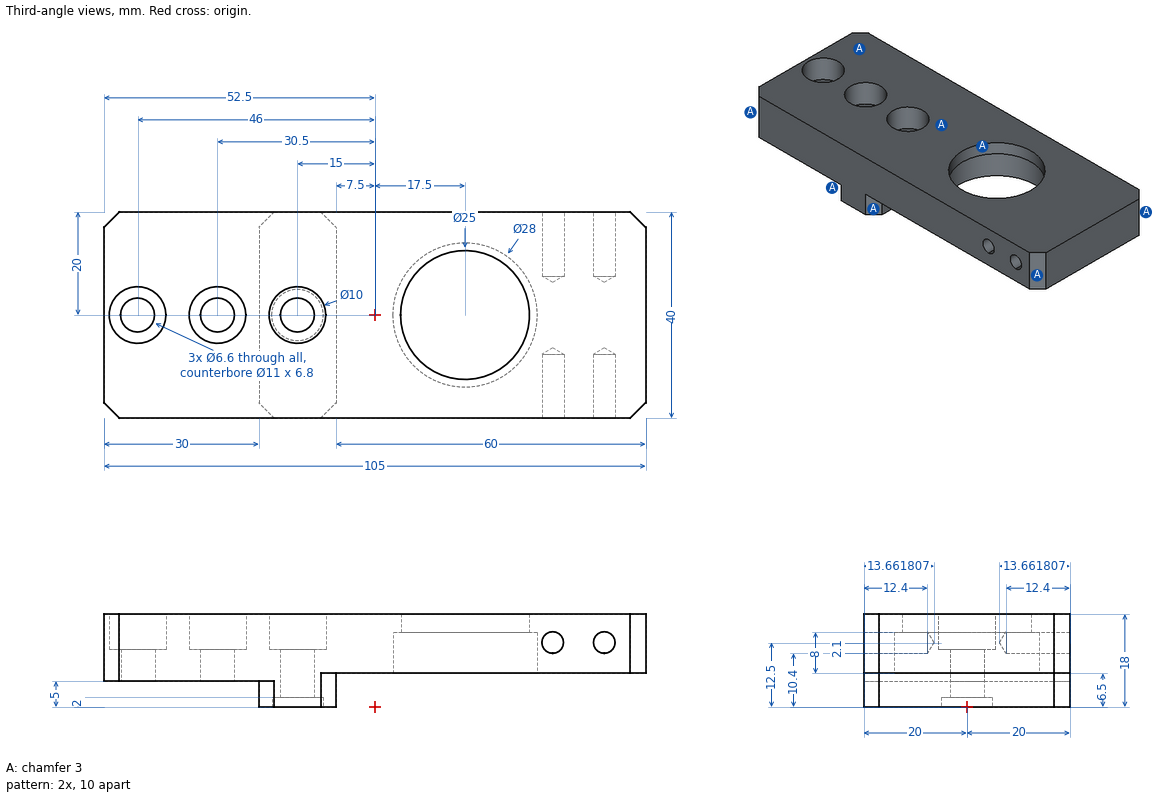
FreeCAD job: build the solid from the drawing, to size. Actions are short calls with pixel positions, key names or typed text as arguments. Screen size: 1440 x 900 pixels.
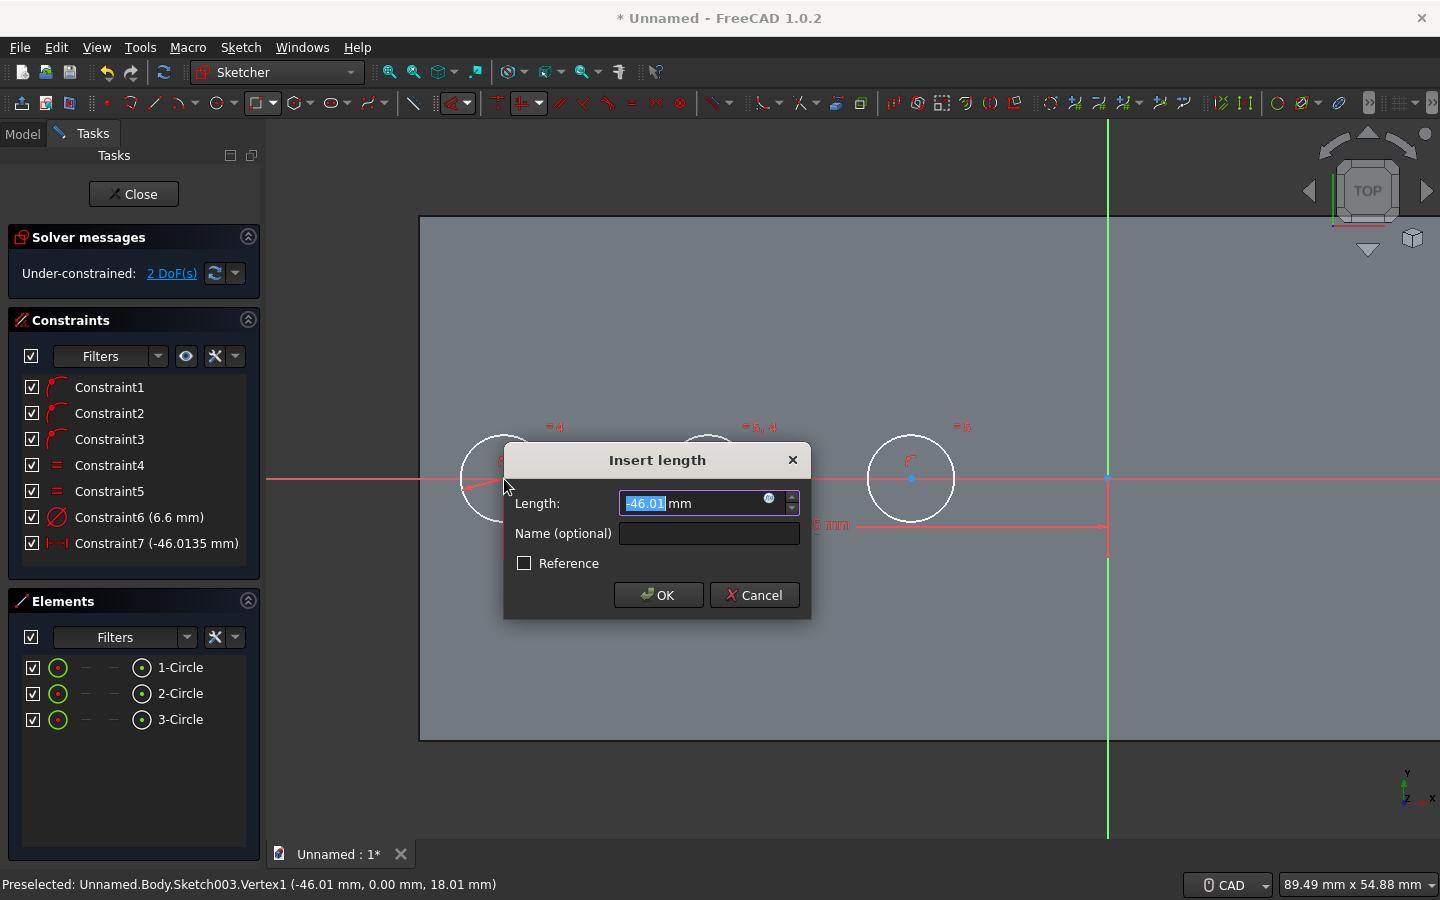
text(-46)
key(Return)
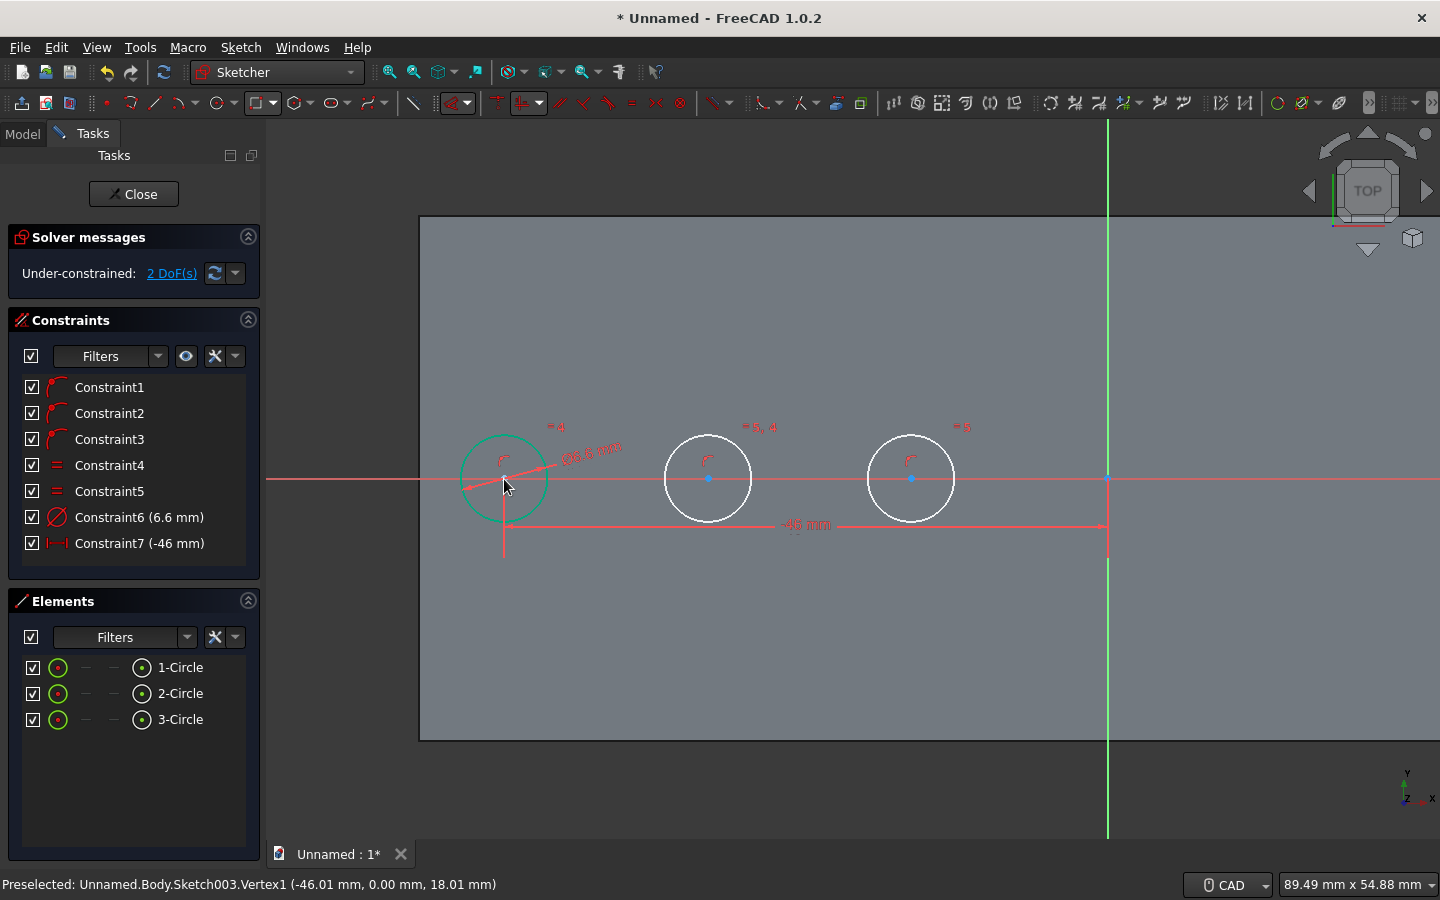
click(911, 479)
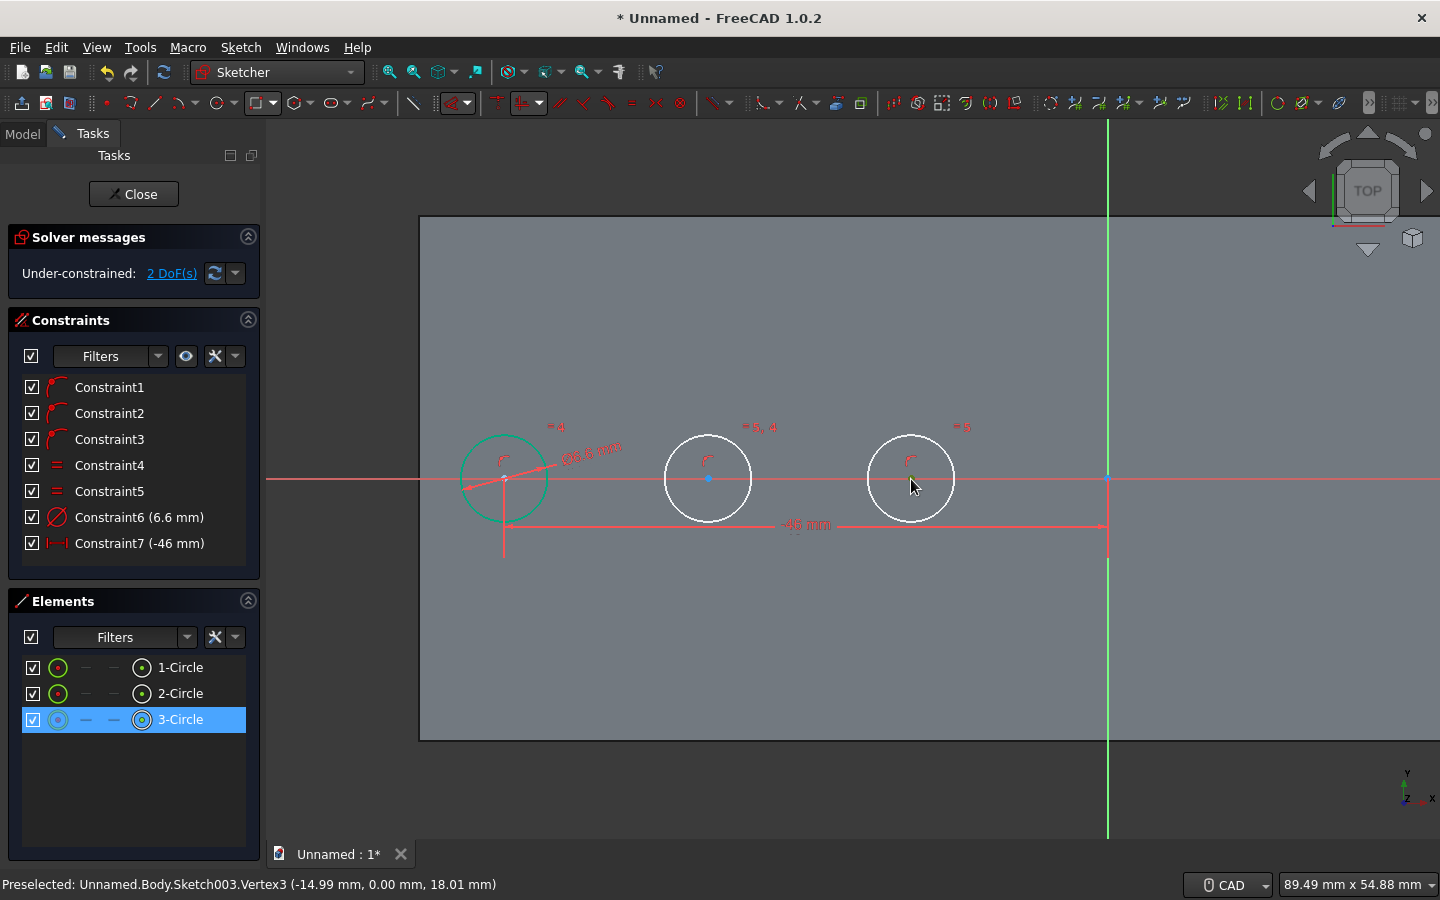
key(l)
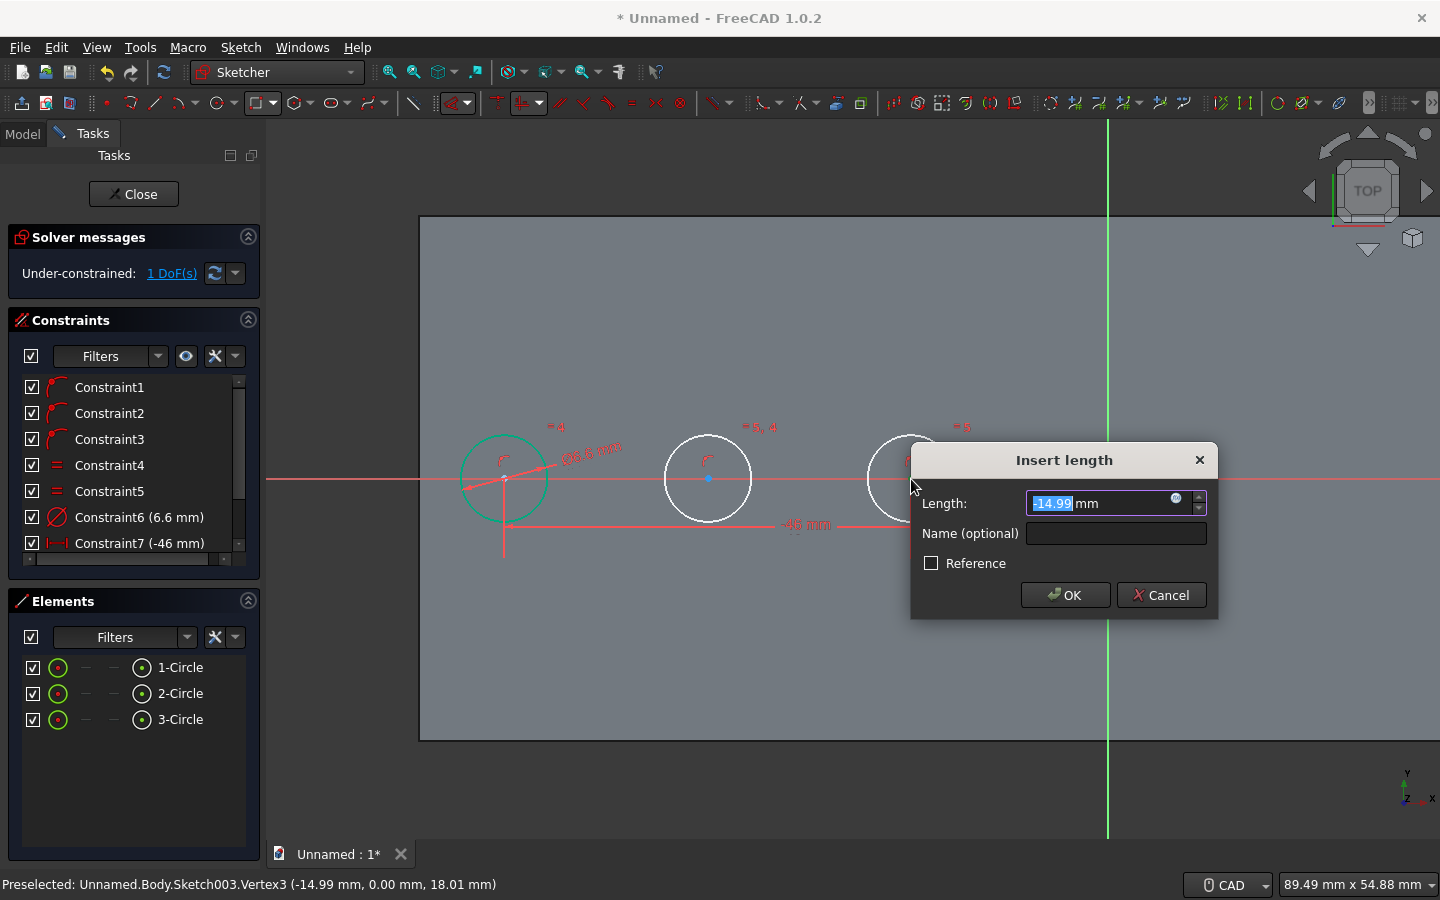
text(-15)
key(Return)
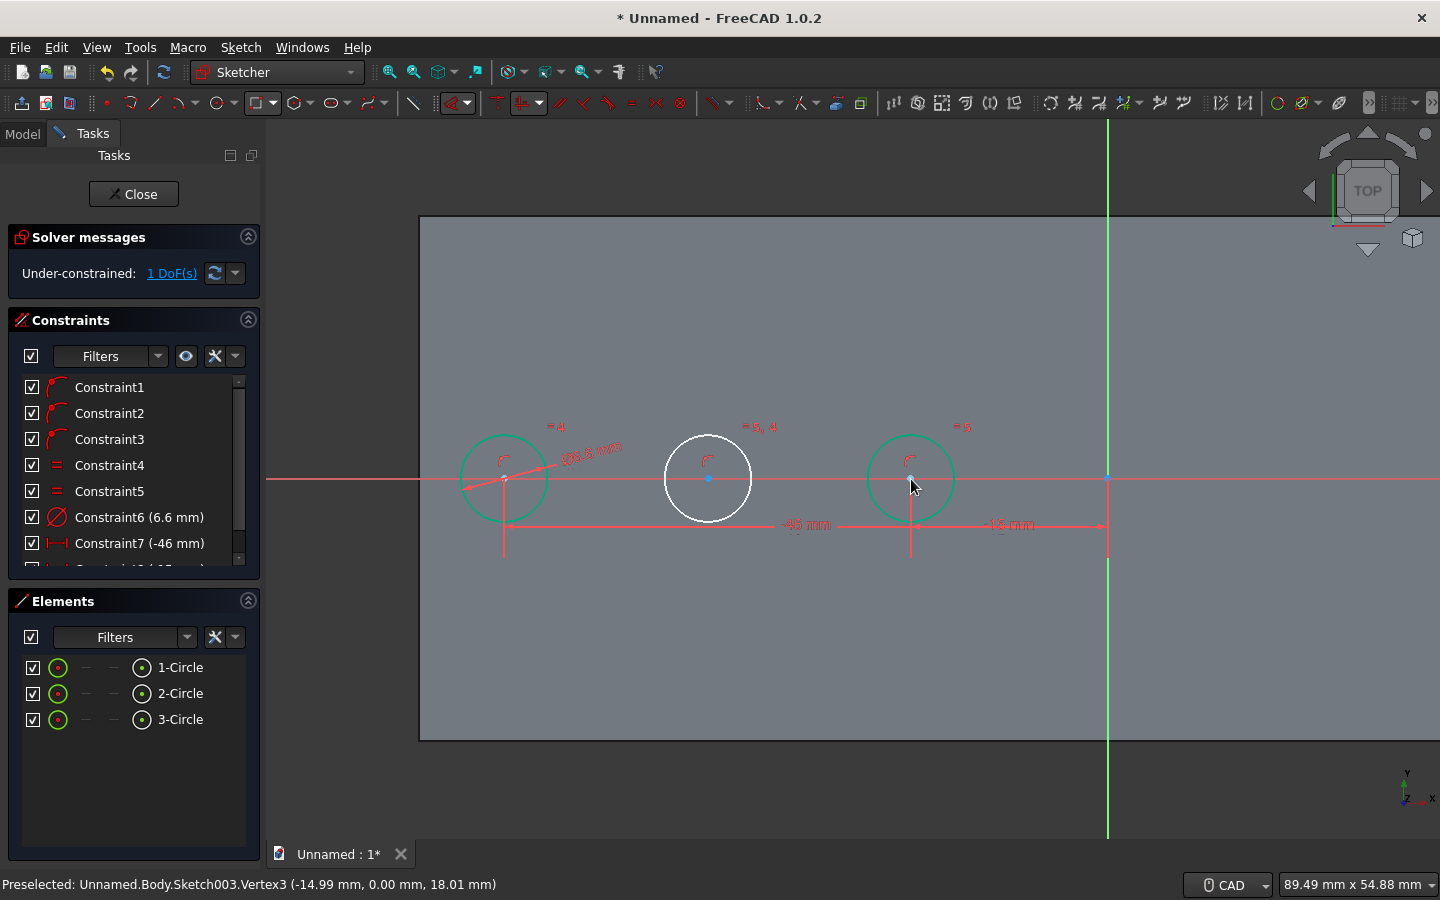
click(708, 479)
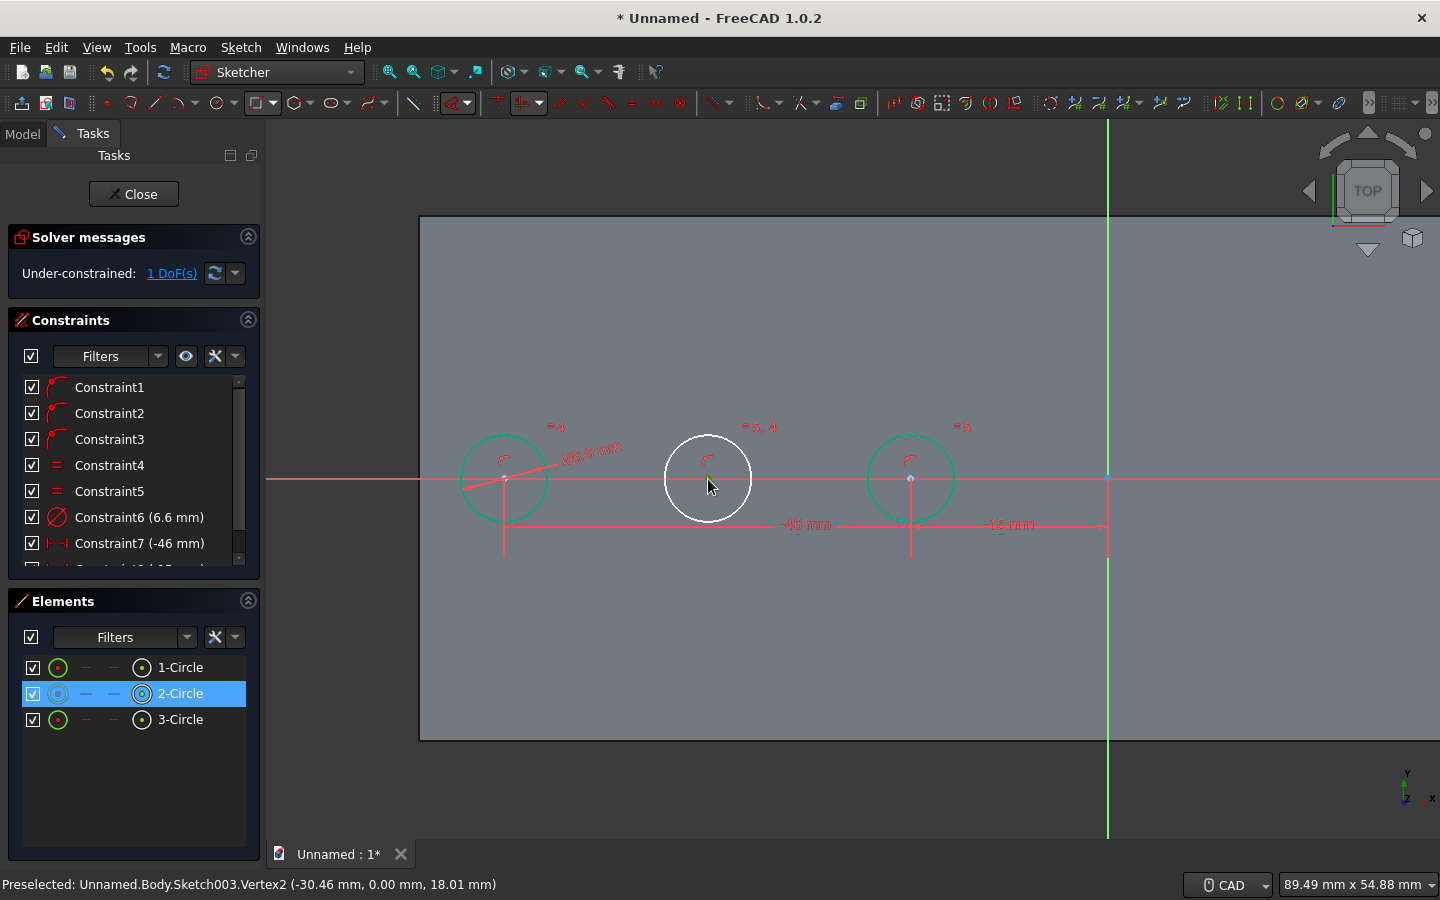
click(470, 104)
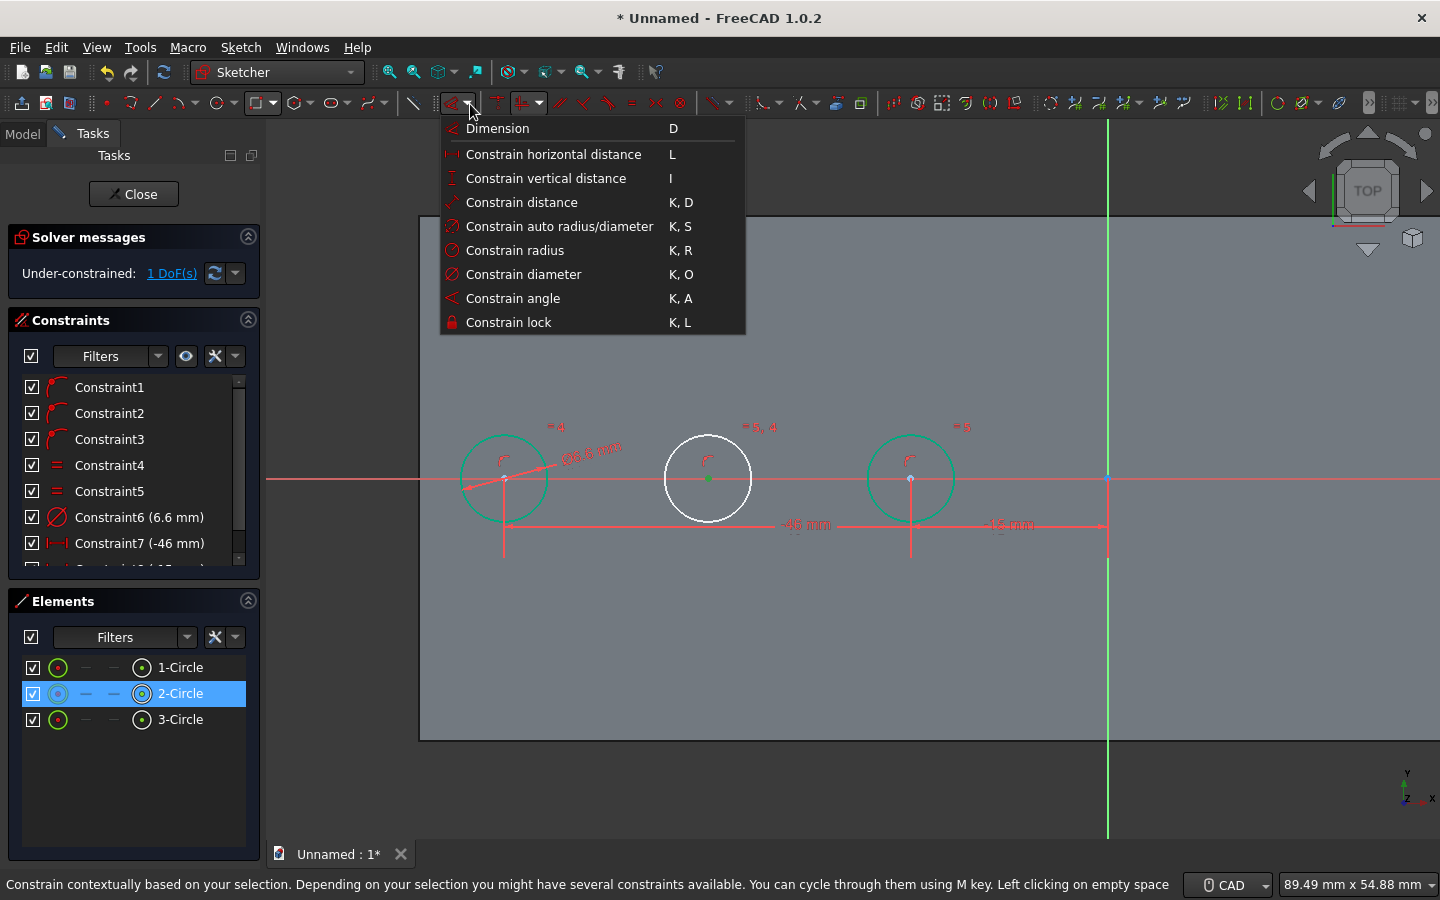
click(593, 154)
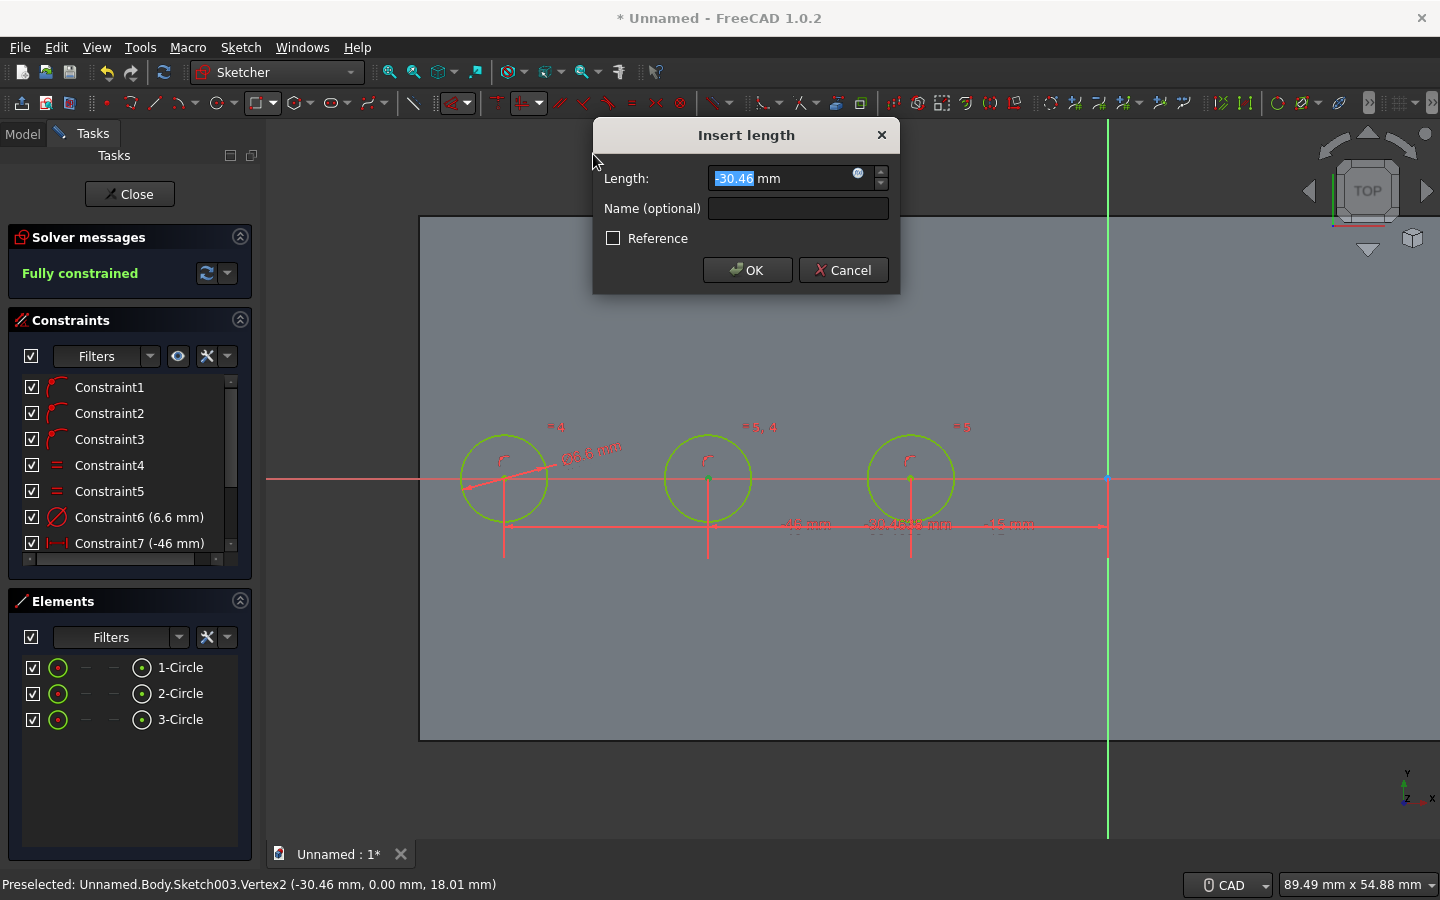
text(-30.5)
key(Return)